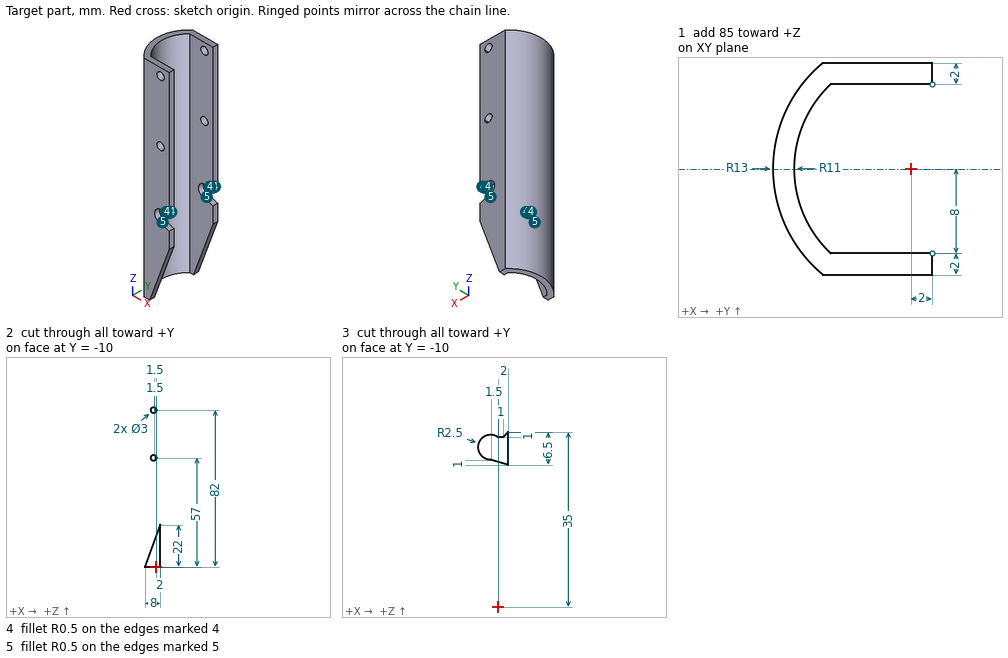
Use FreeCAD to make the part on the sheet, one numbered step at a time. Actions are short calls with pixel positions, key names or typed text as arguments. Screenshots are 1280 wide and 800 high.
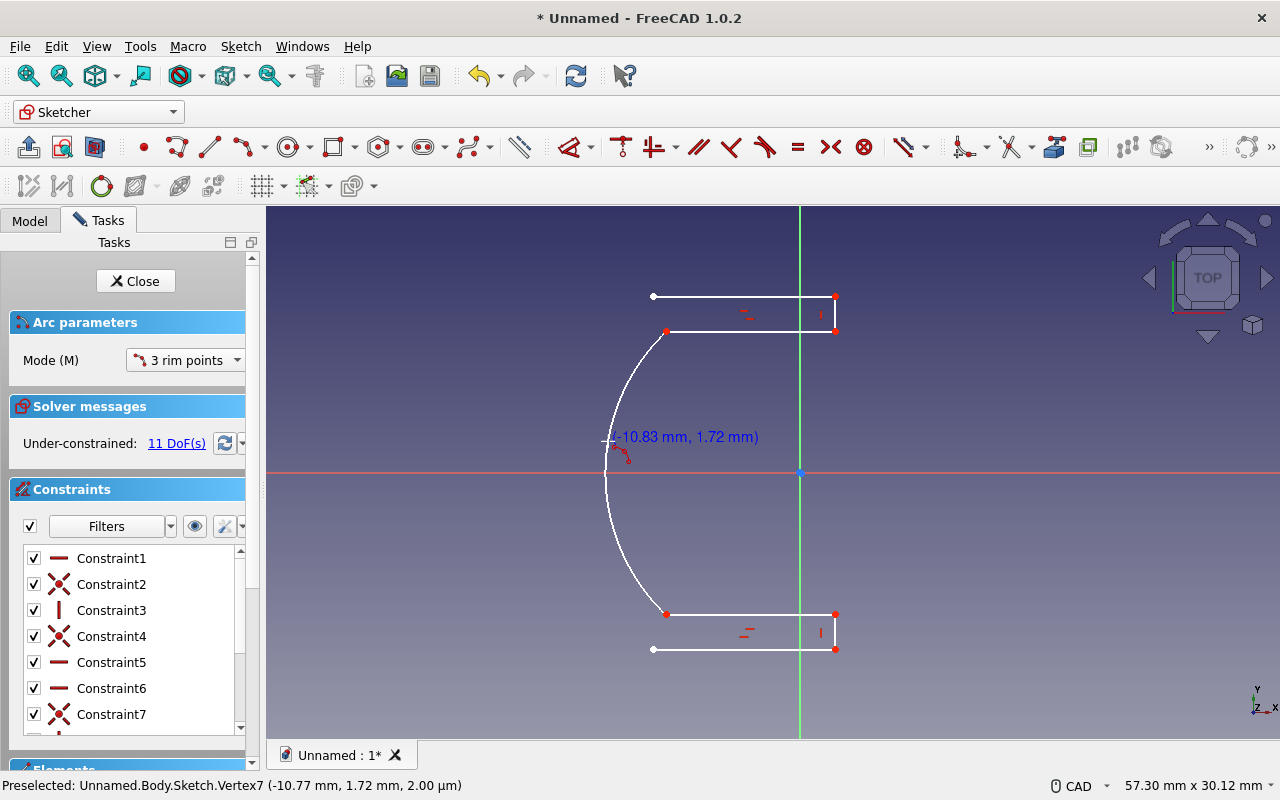
click(653, 297)
click(653, 650)
click(573, 432)
key(Escape)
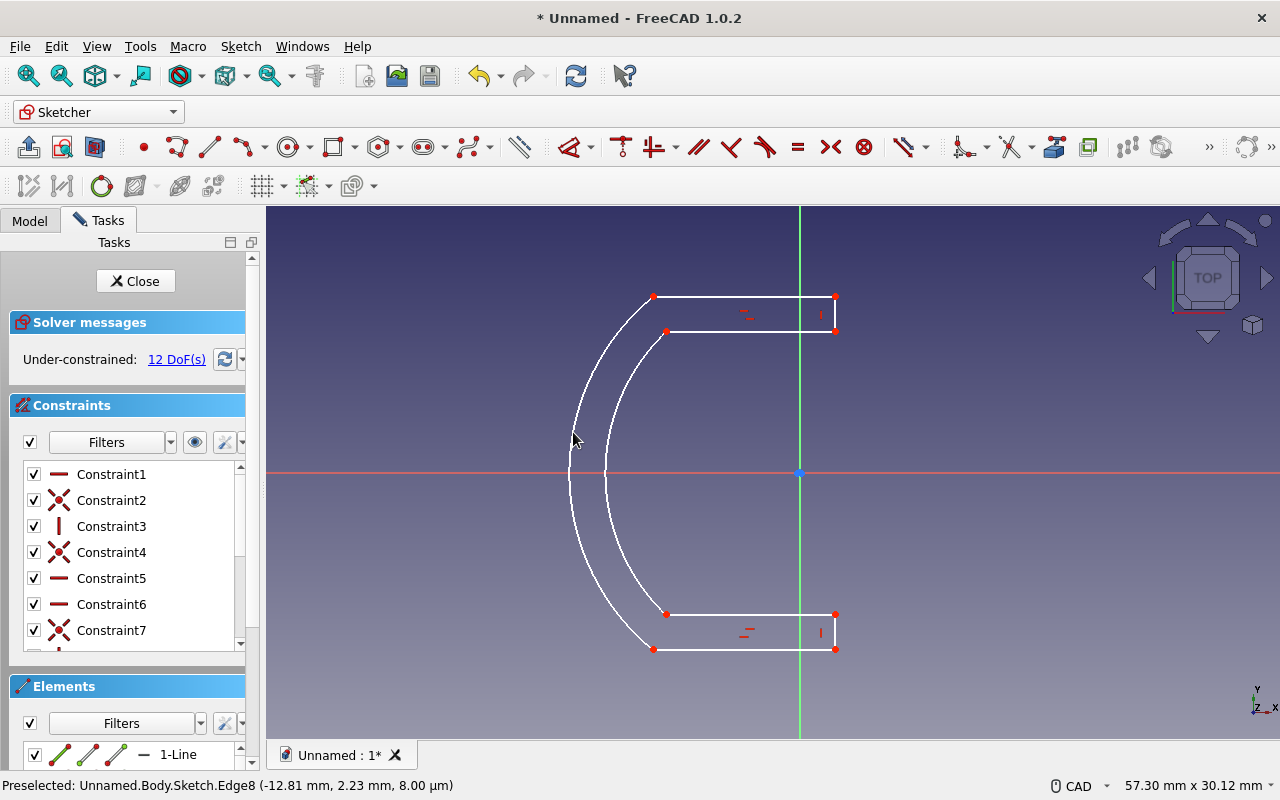
click(616, 411)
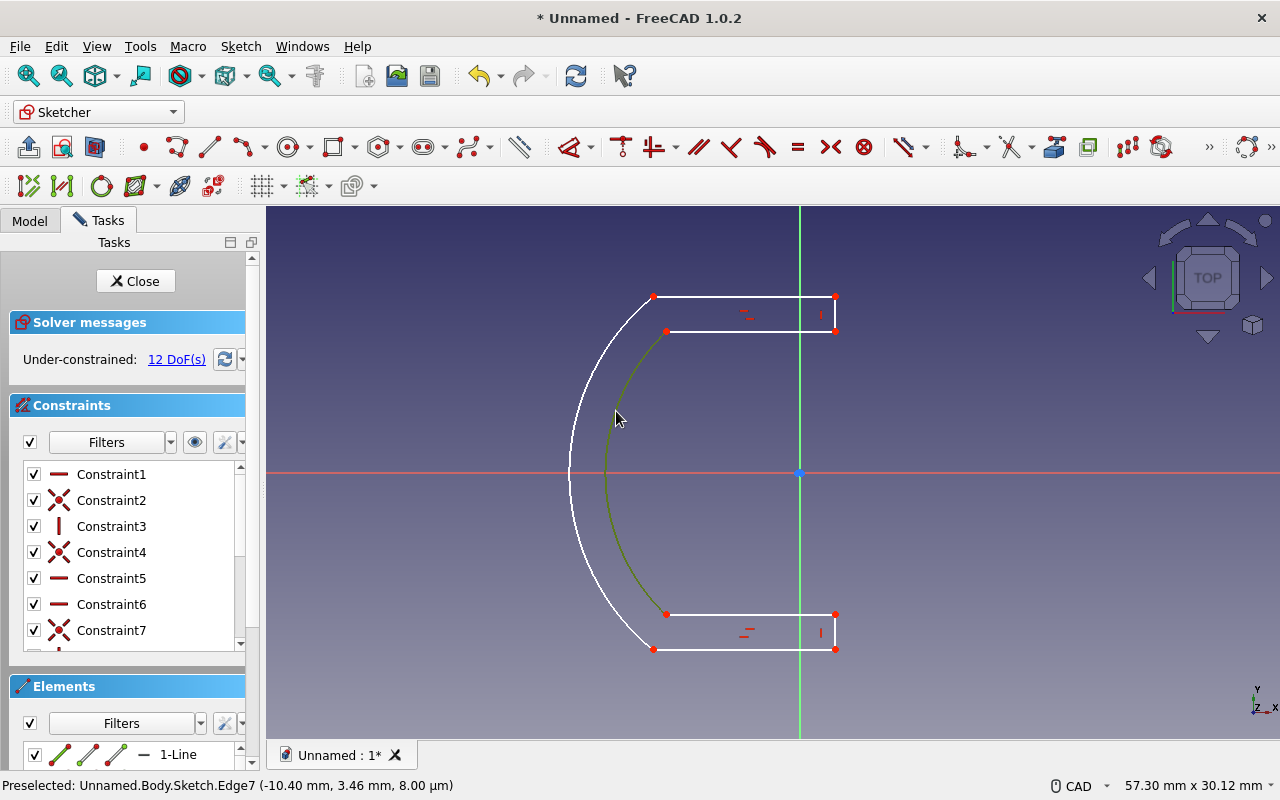
click(584, 394)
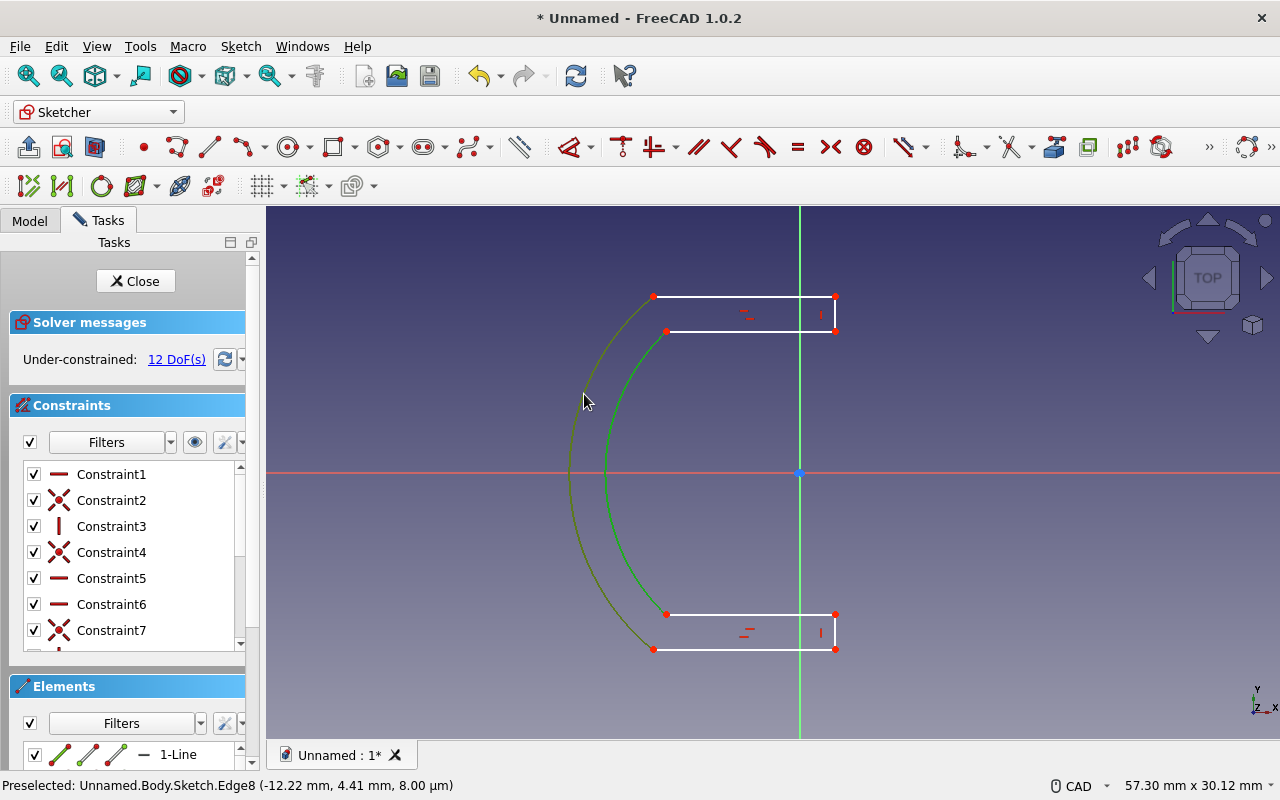
click(621, 148)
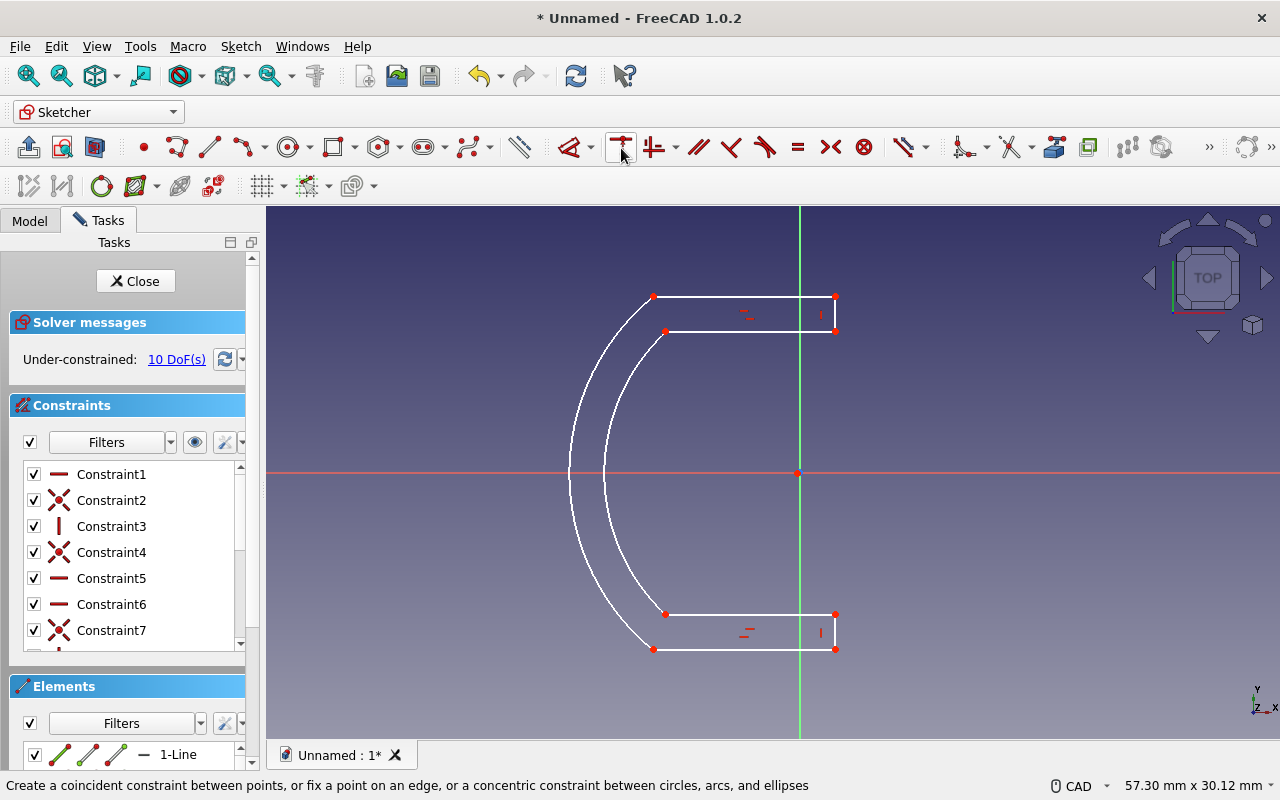
drag(787, 462, 810, 483)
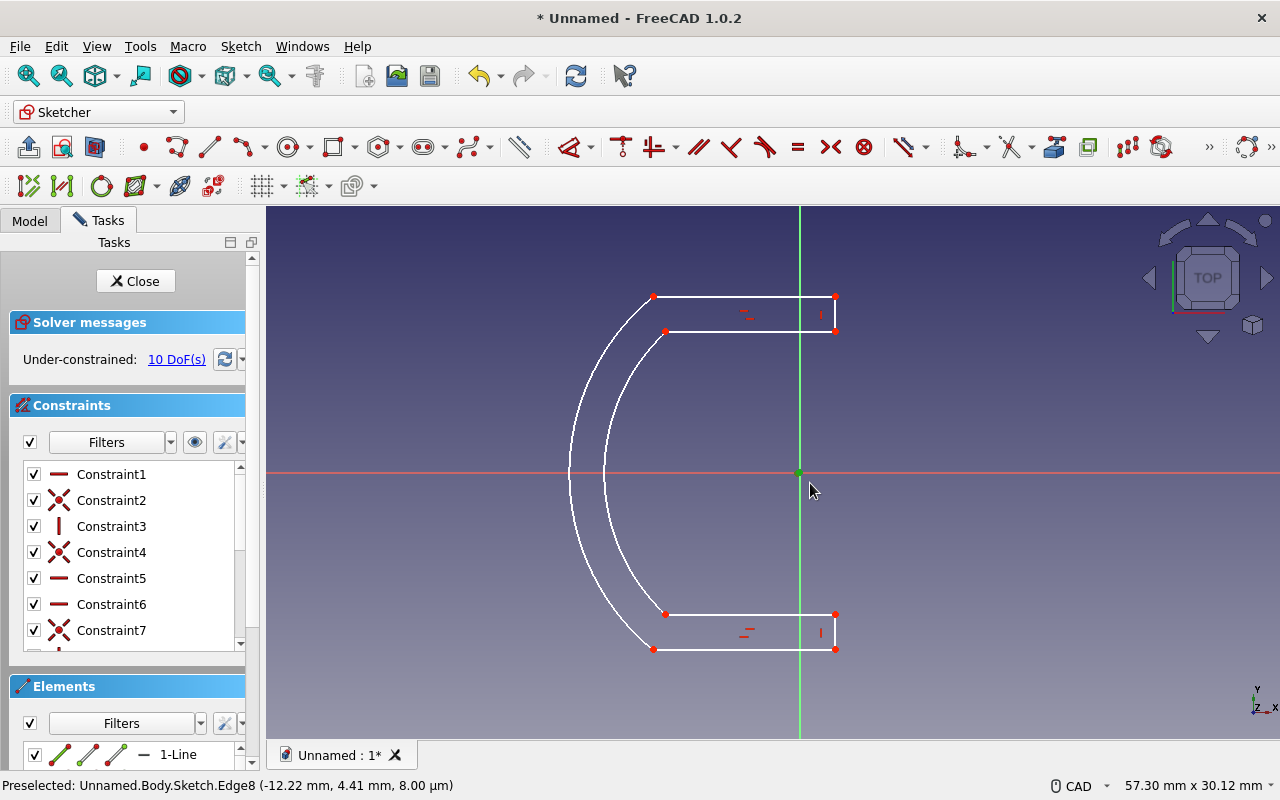
click(621, 148)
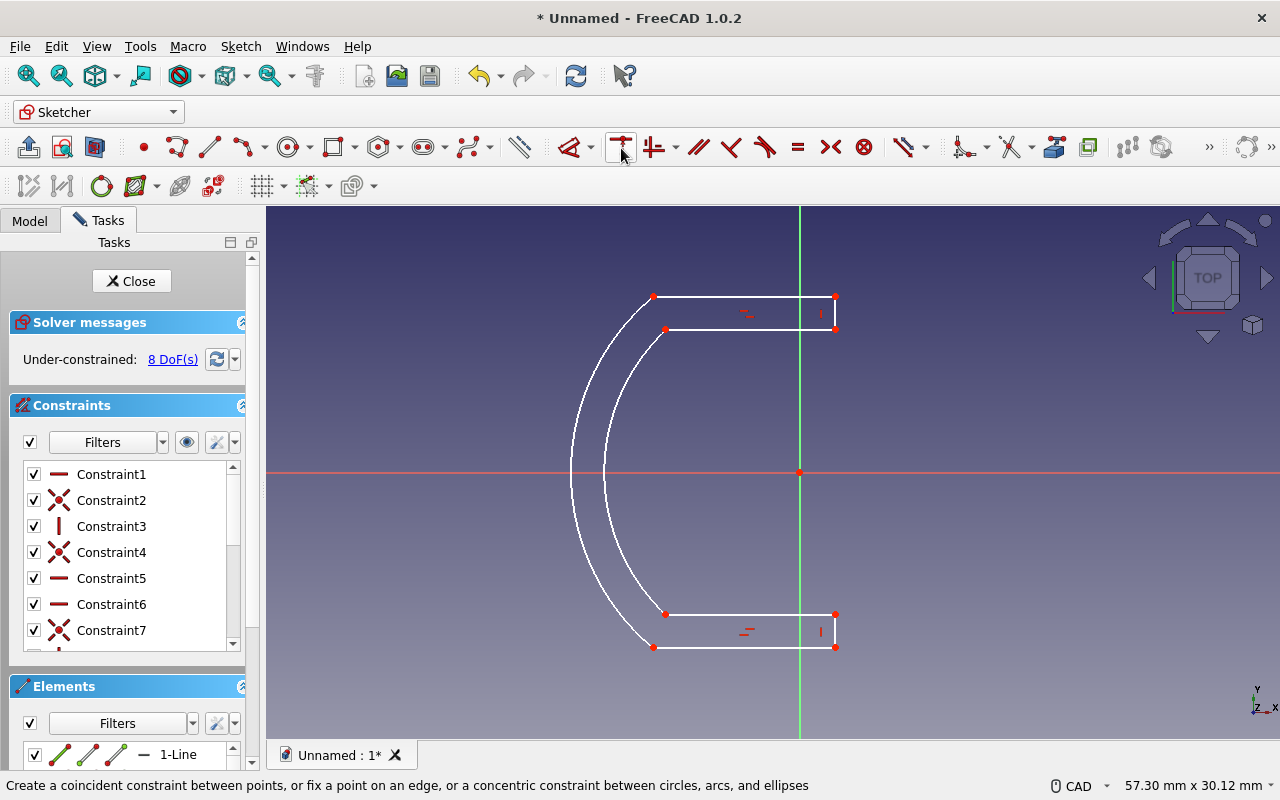
click(835, 615)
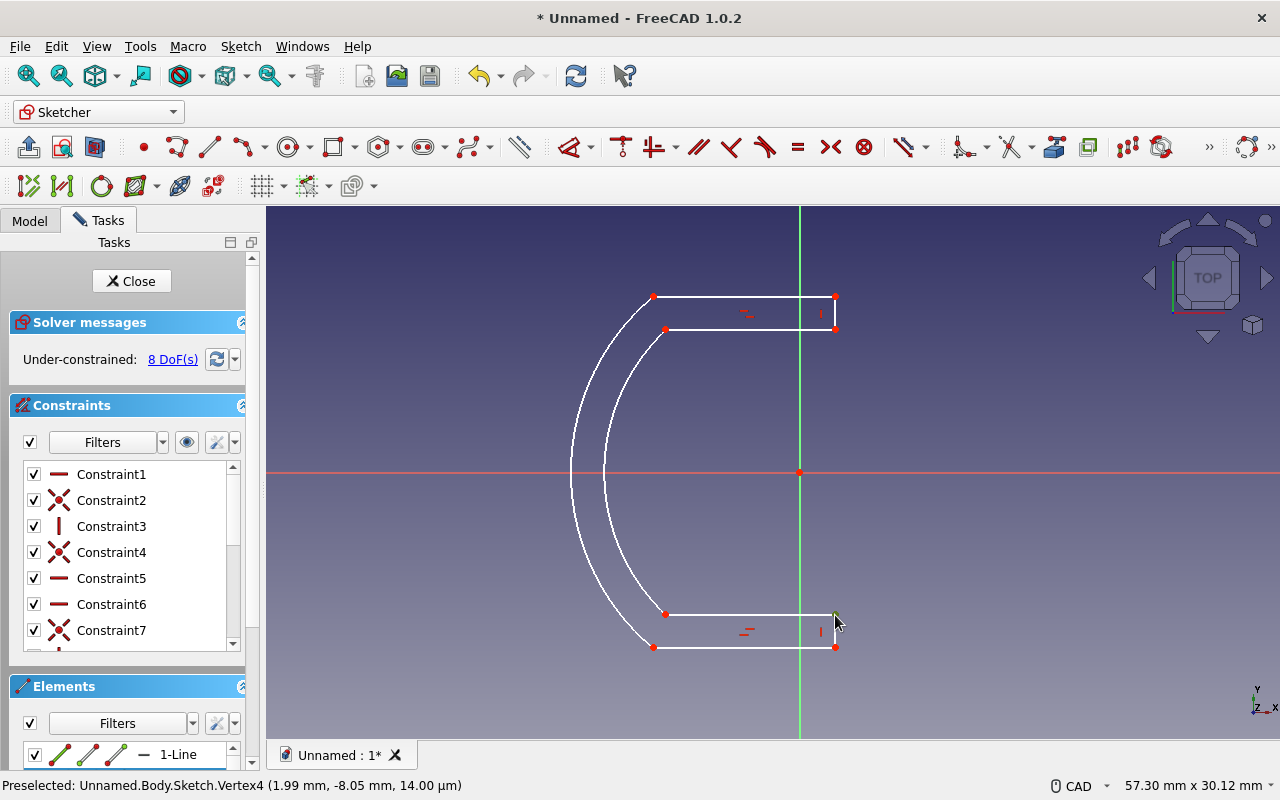
click(835, 330)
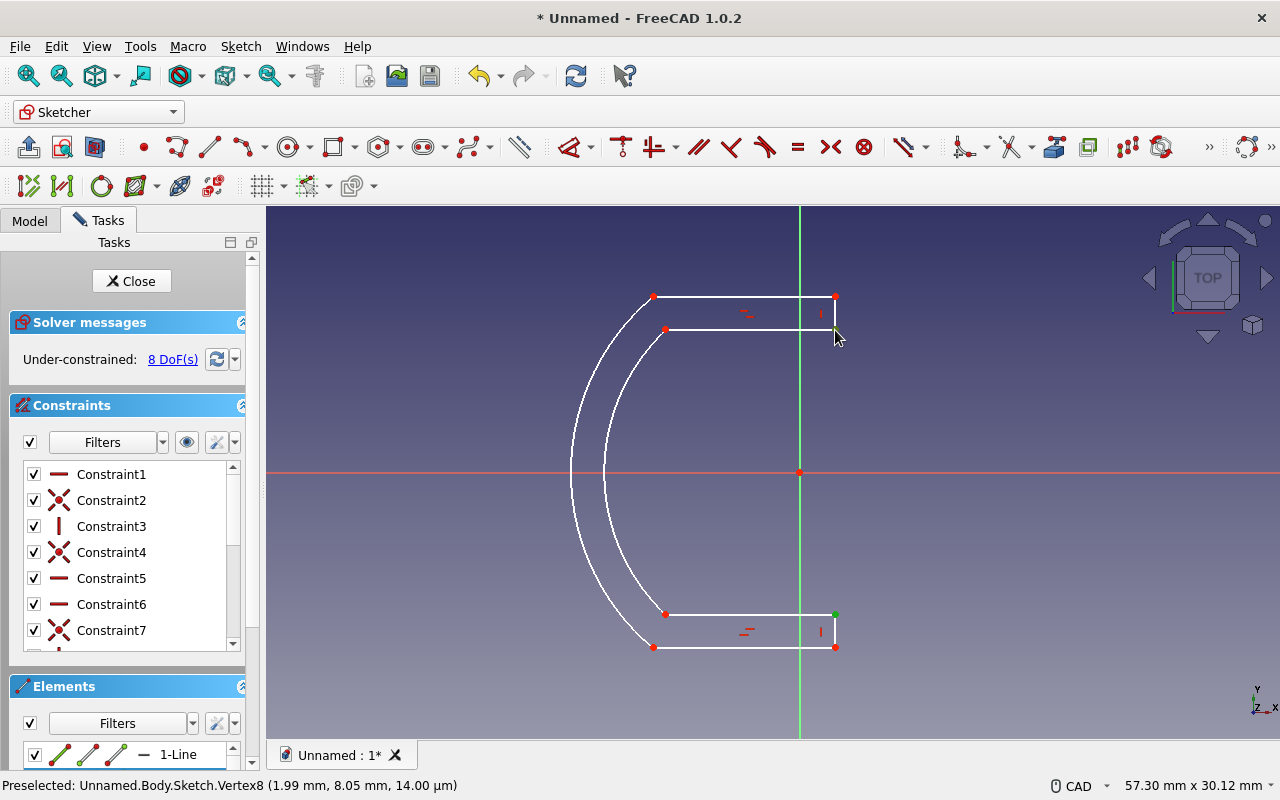
click(353, 472)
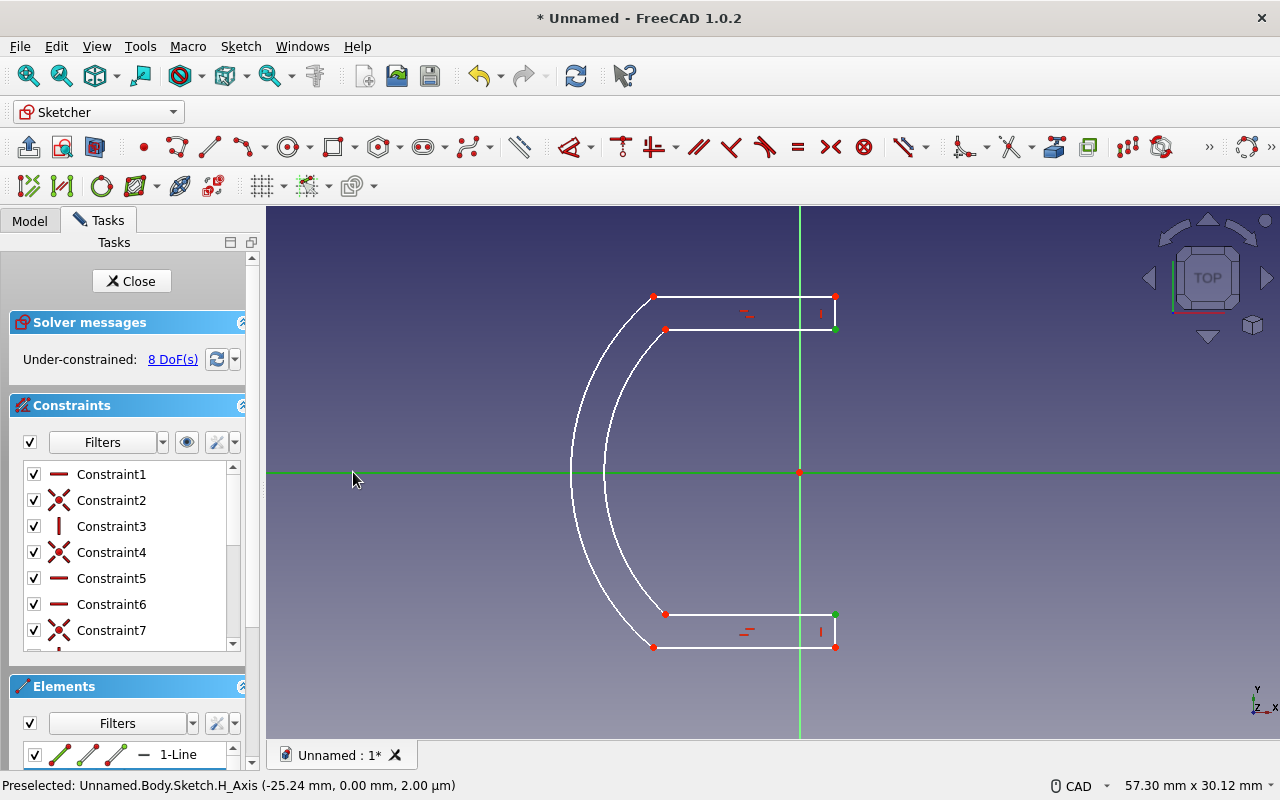
click(831, 148)